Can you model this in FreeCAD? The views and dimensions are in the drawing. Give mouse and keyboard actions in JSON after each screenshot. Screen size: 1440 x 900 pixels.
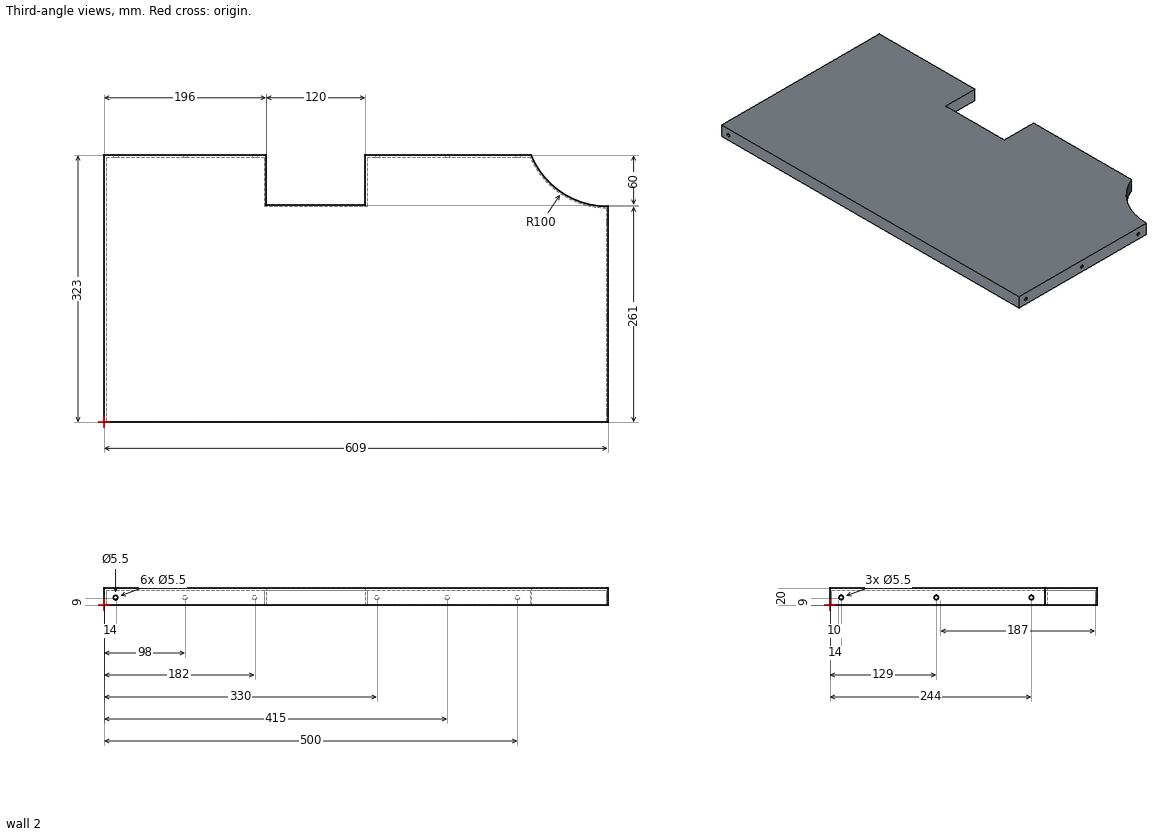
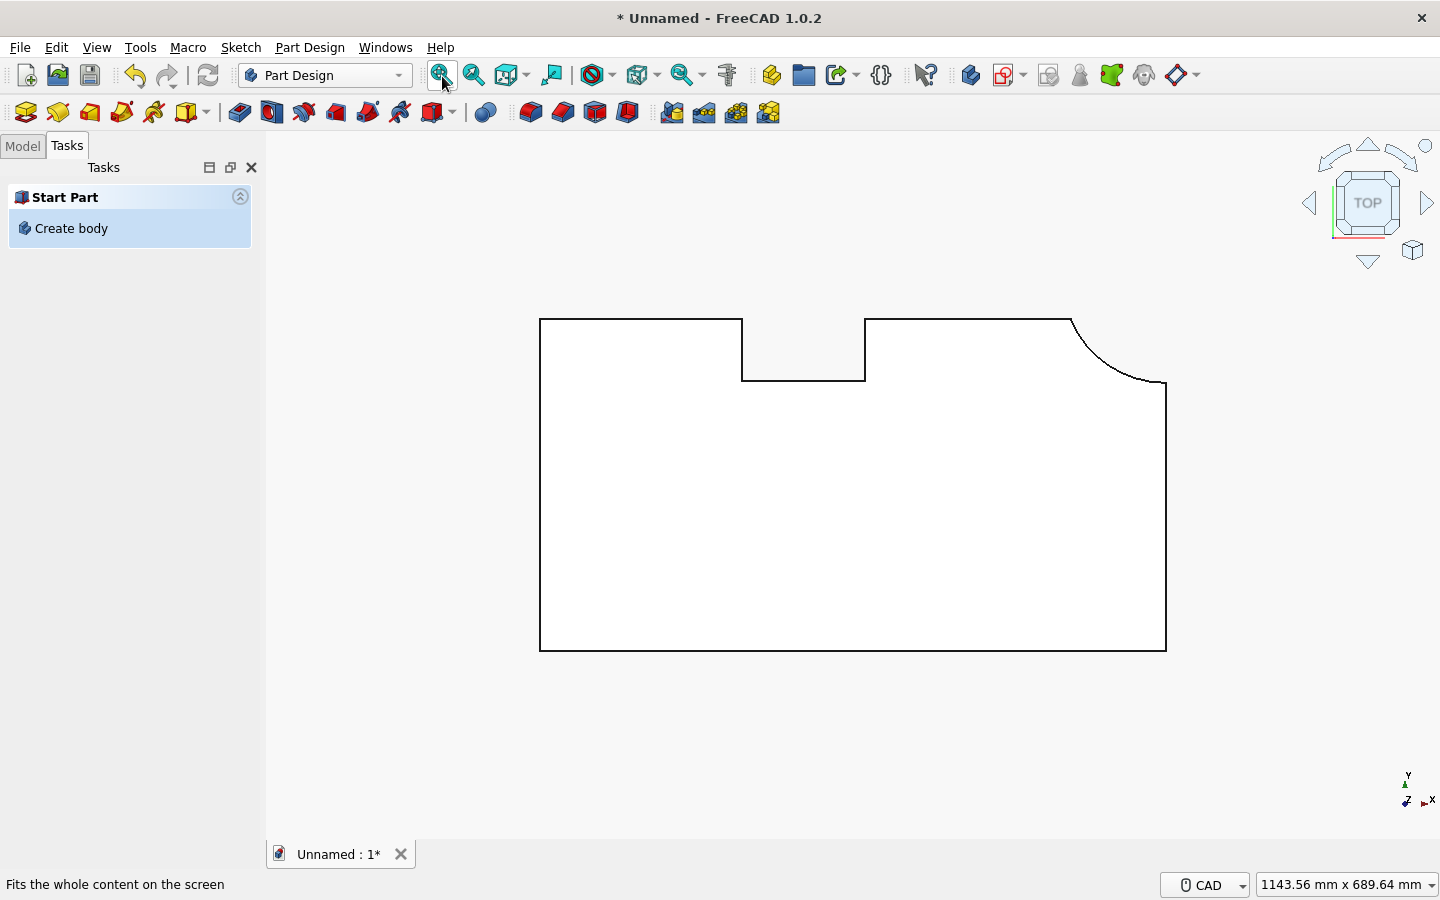
{"action": "key", "text": "1"}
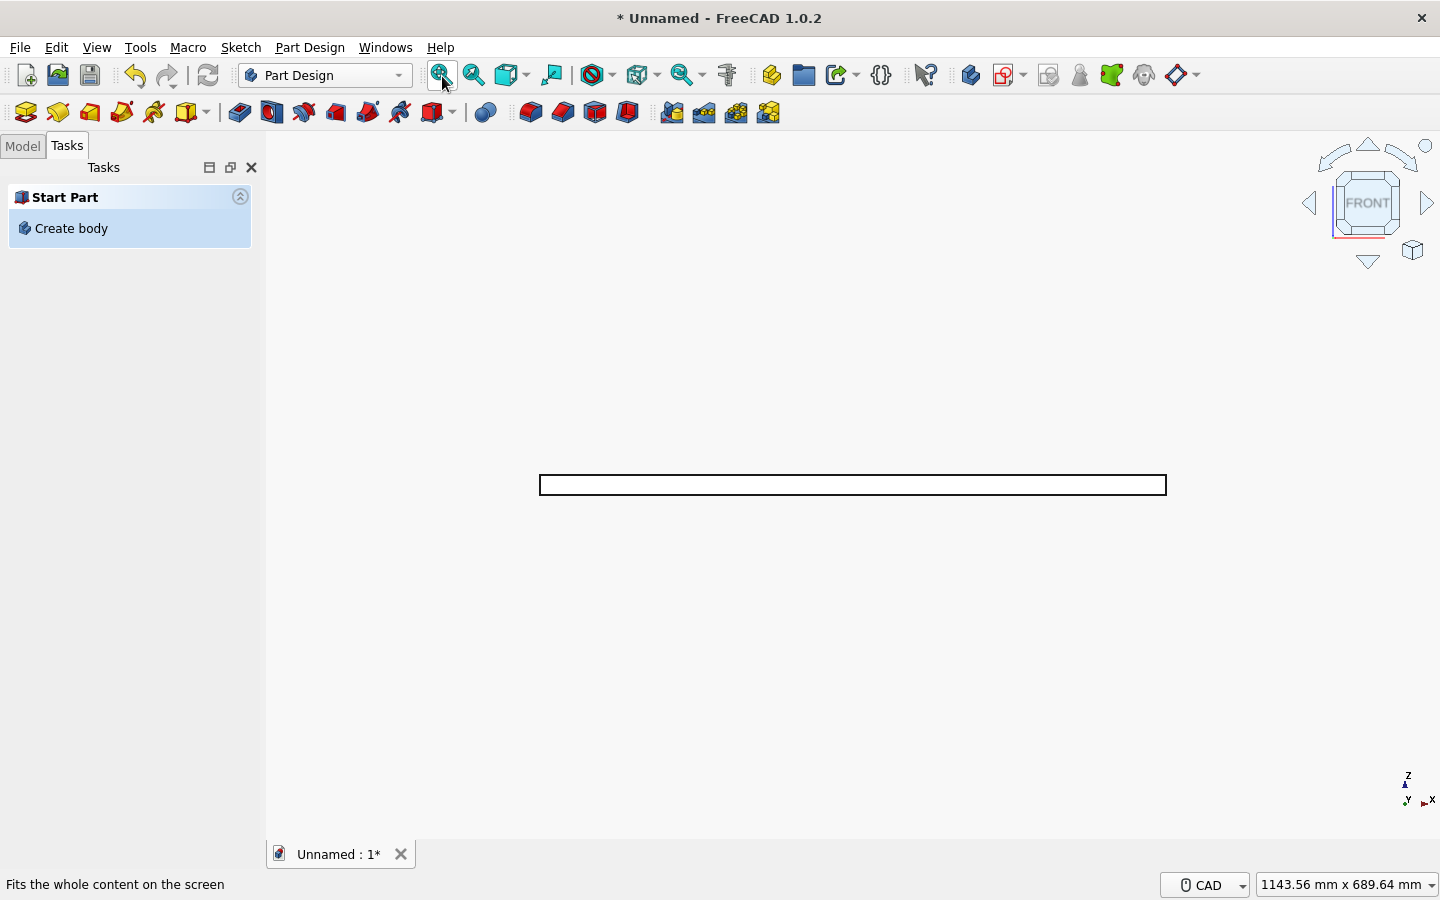
{"action": "key", "text": "3"}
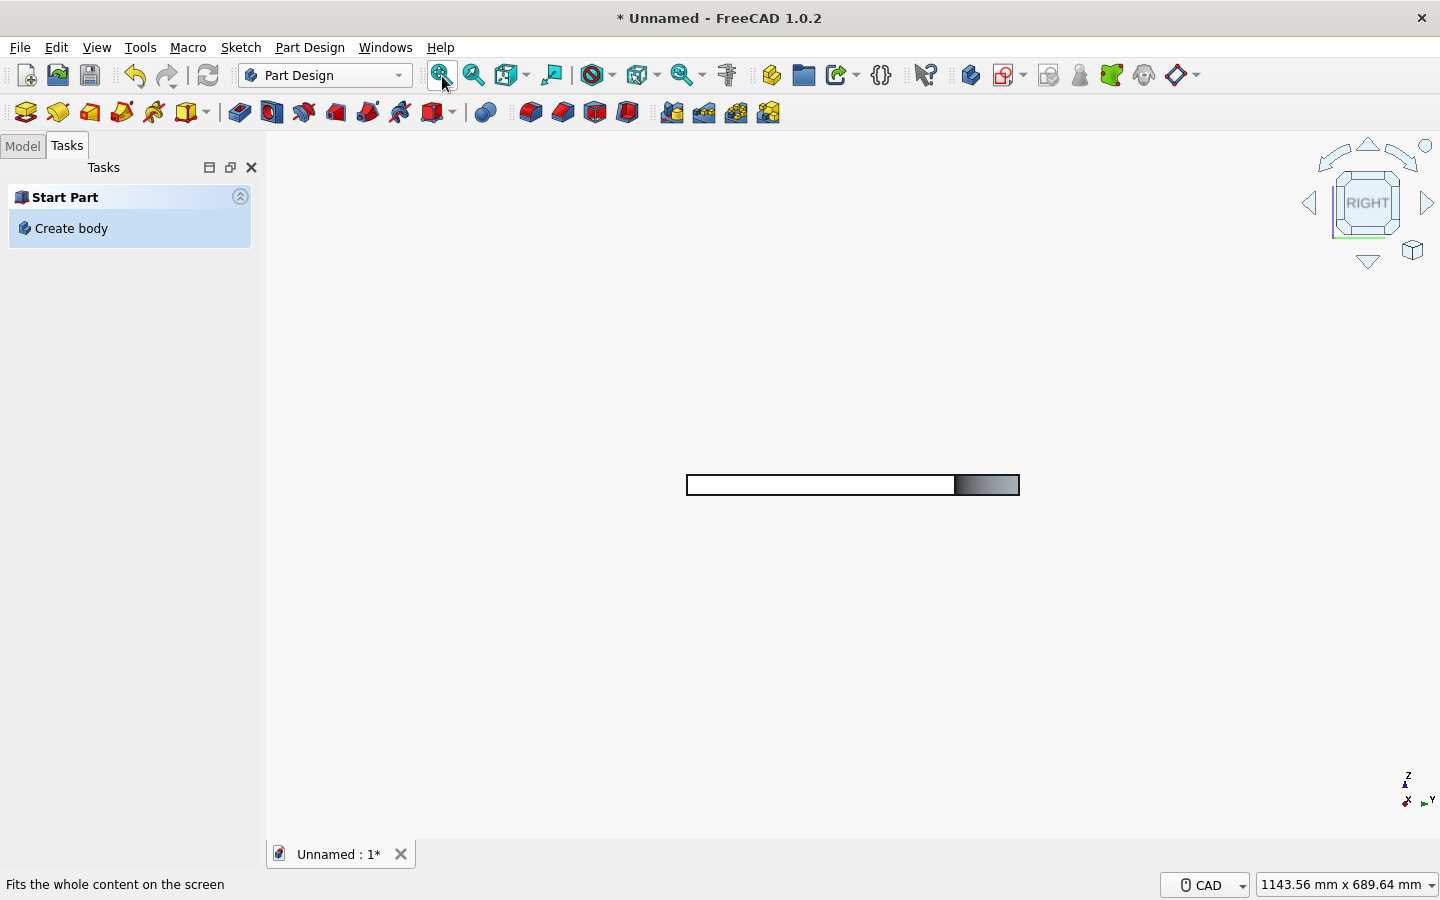
{"action": "left_click", "coordinate": [442, 76]}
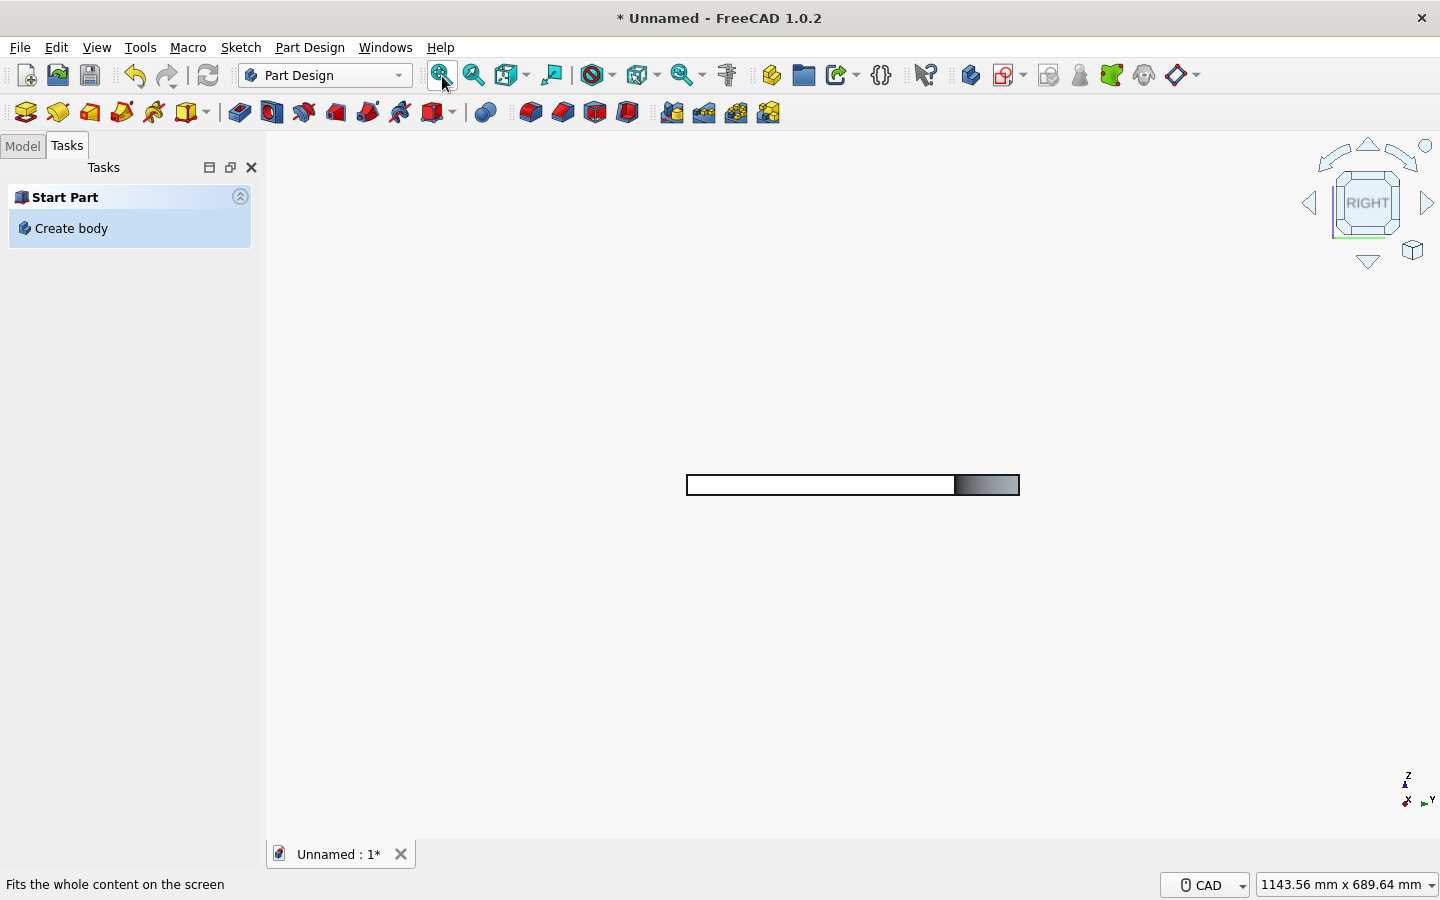
{"action": "key", "text": "5"}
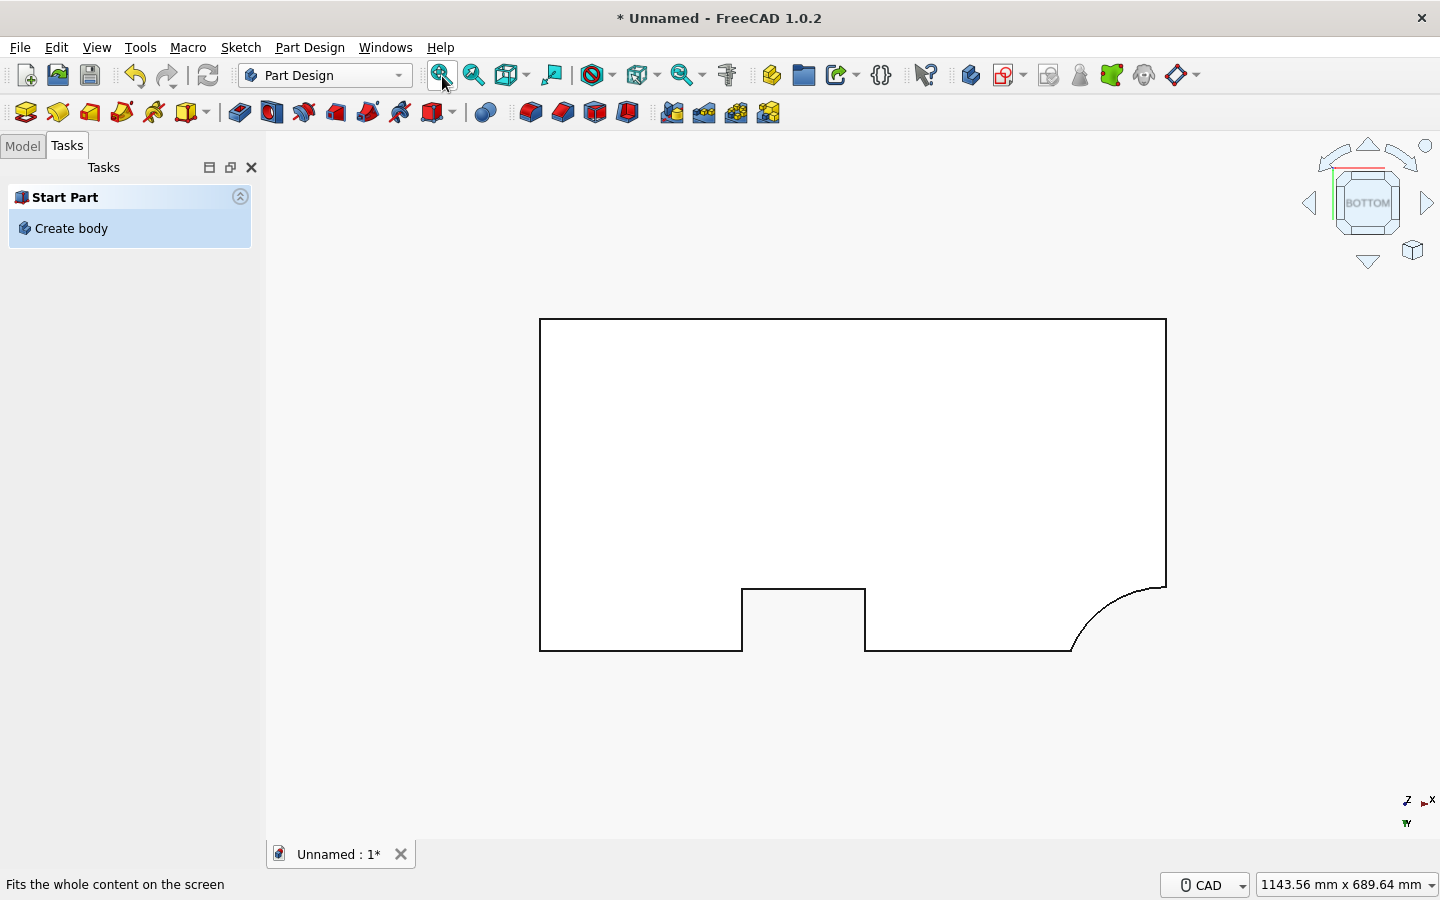
{"action": "left_click", "coordinate": [1032, 484]}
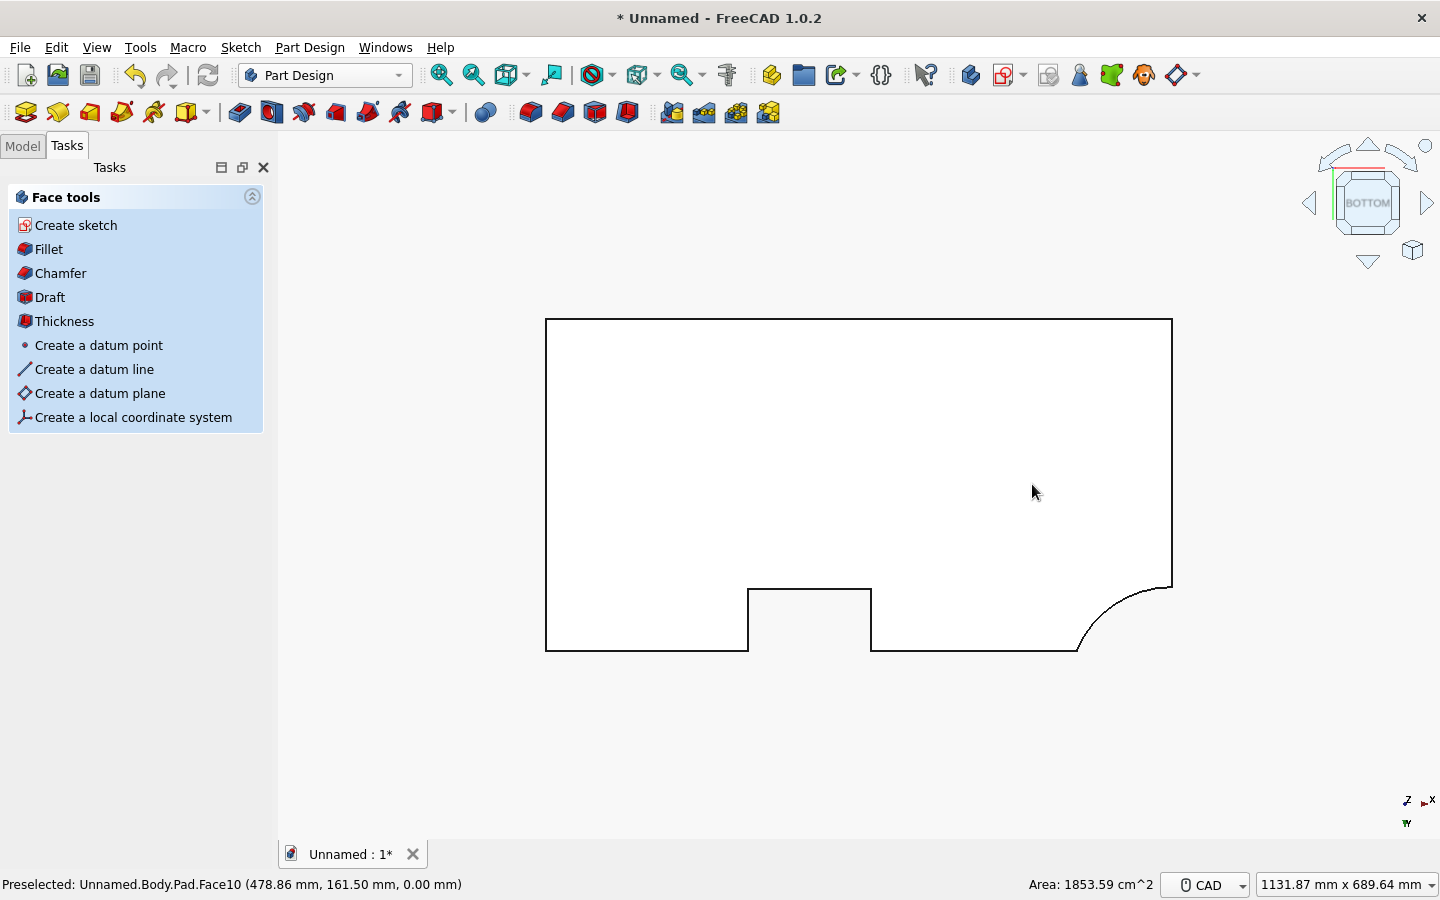
{"action": "left_click", "coordinate": [628, 112]}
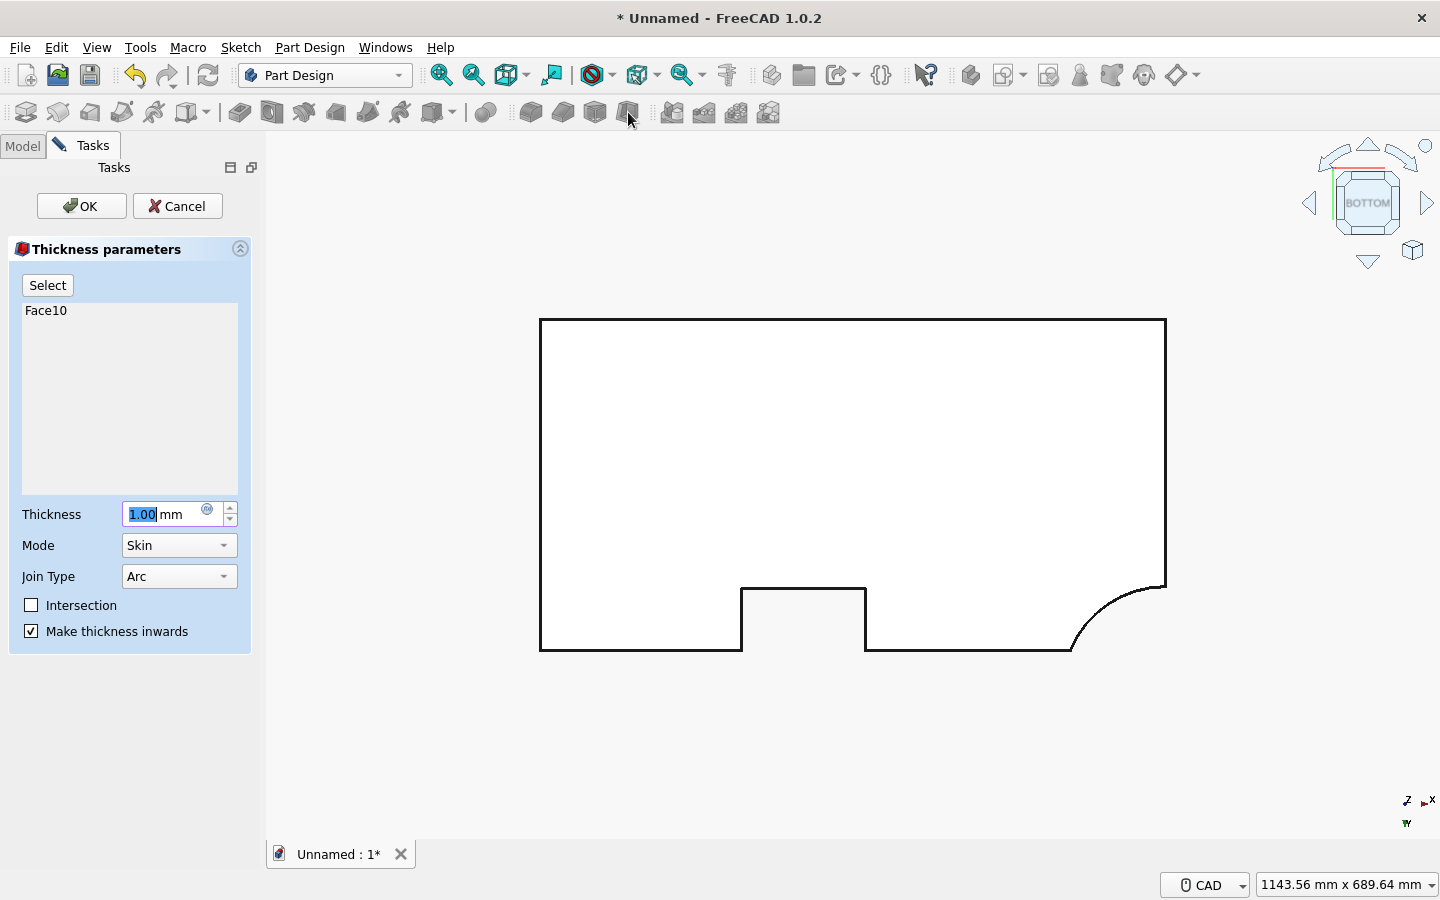
{"action": "type", "text": "2"}
{"action": "key", "text": "Tab"}